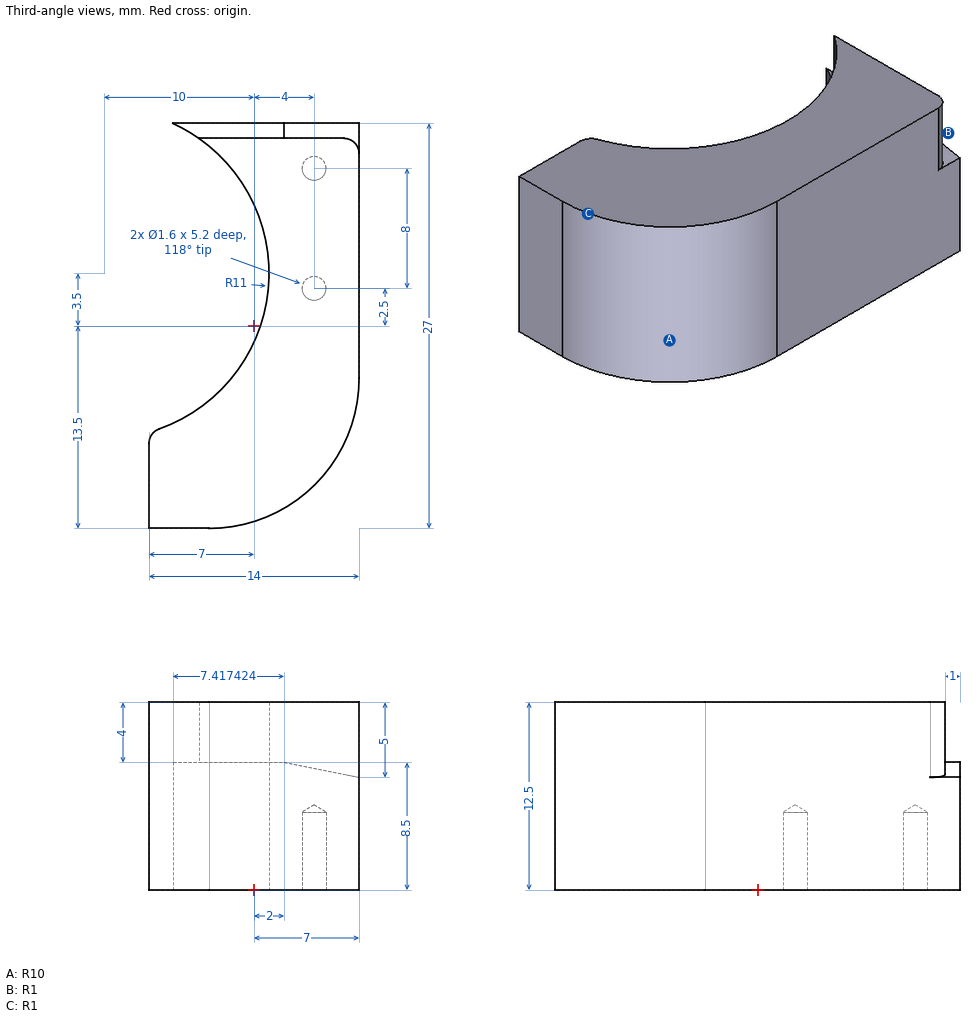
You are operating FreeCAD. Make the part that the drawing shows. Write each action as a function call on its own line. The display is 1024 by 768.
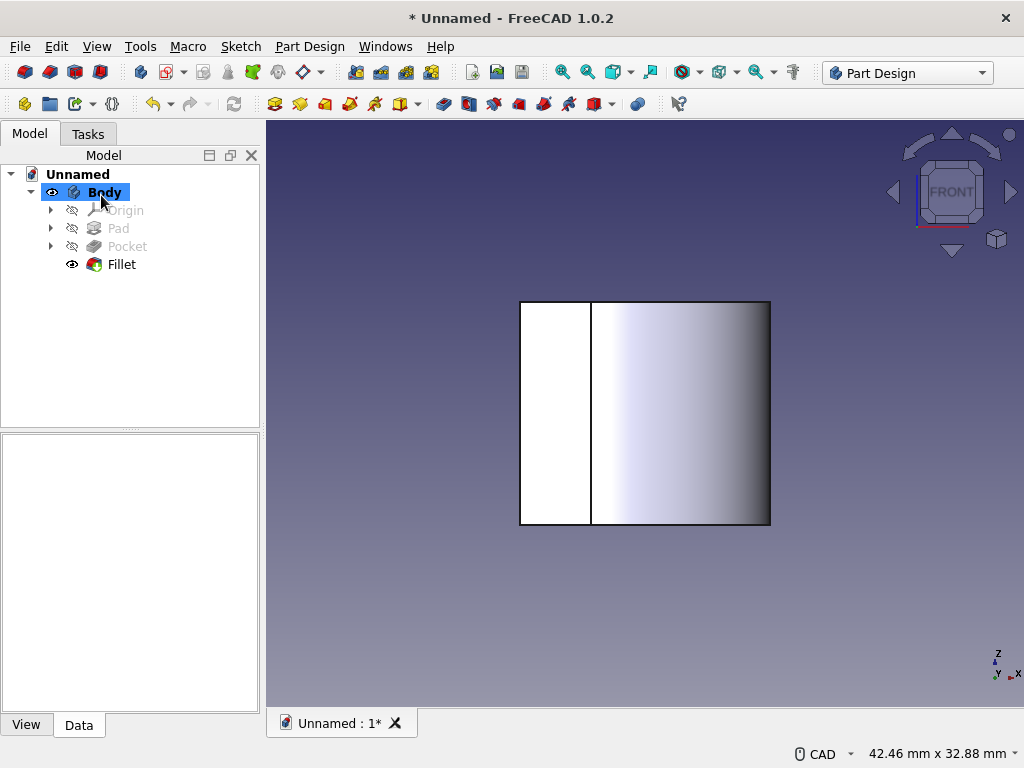
click(563, 72)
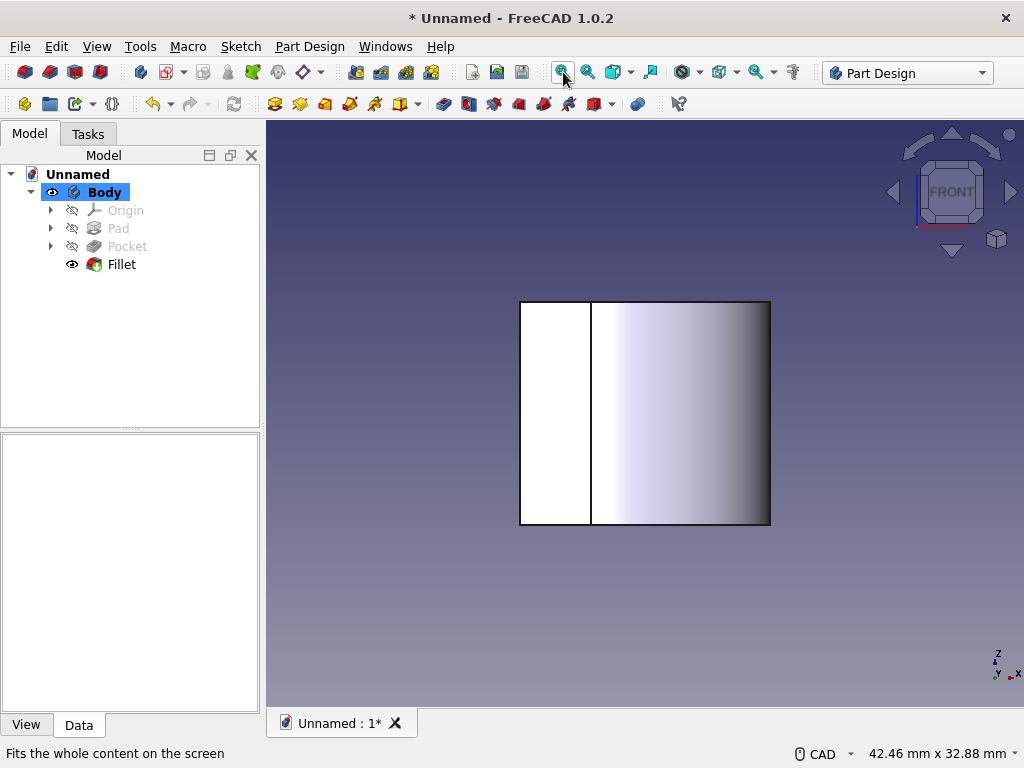
key(3)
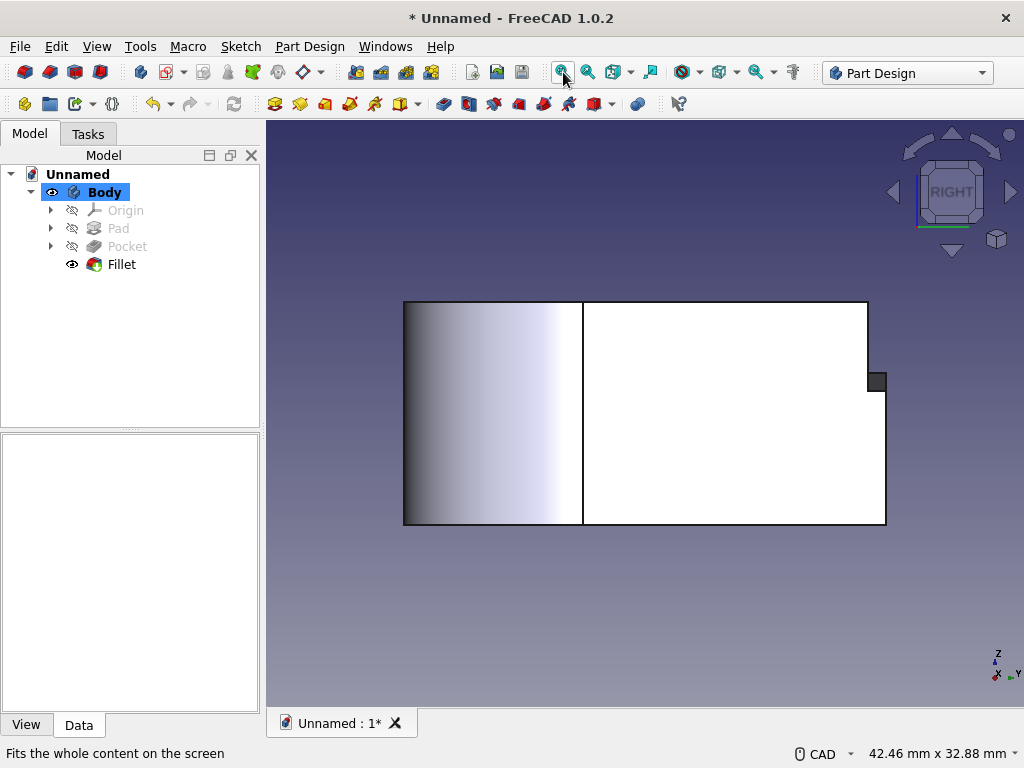
click(868, 346)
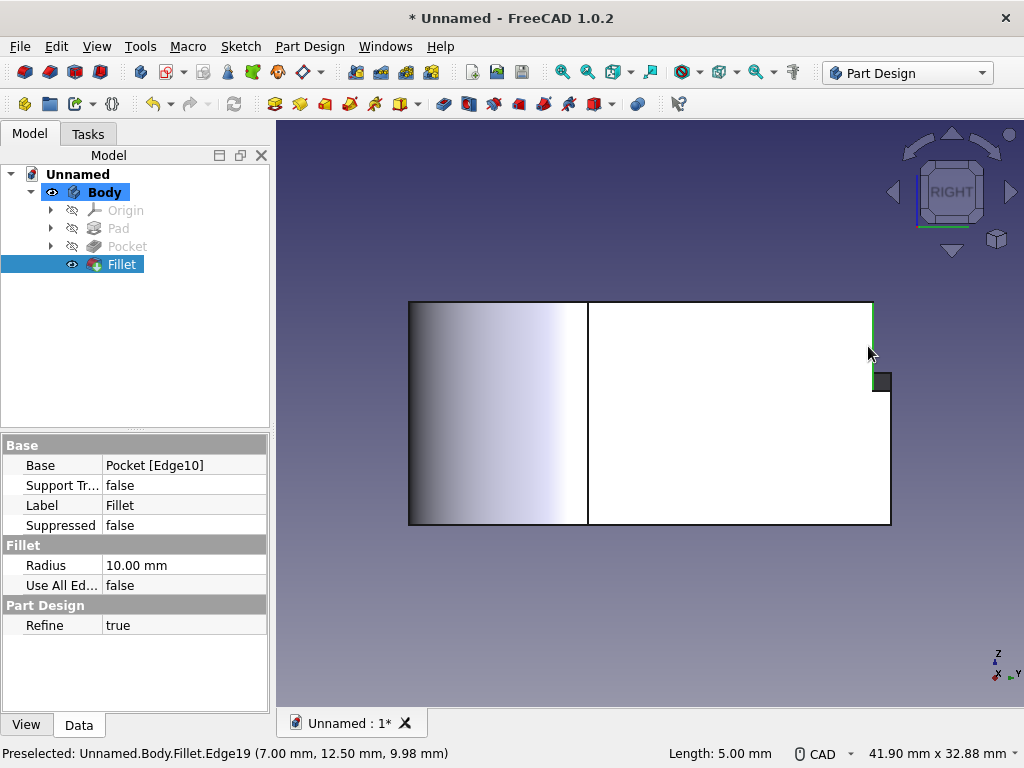
click(25, 72)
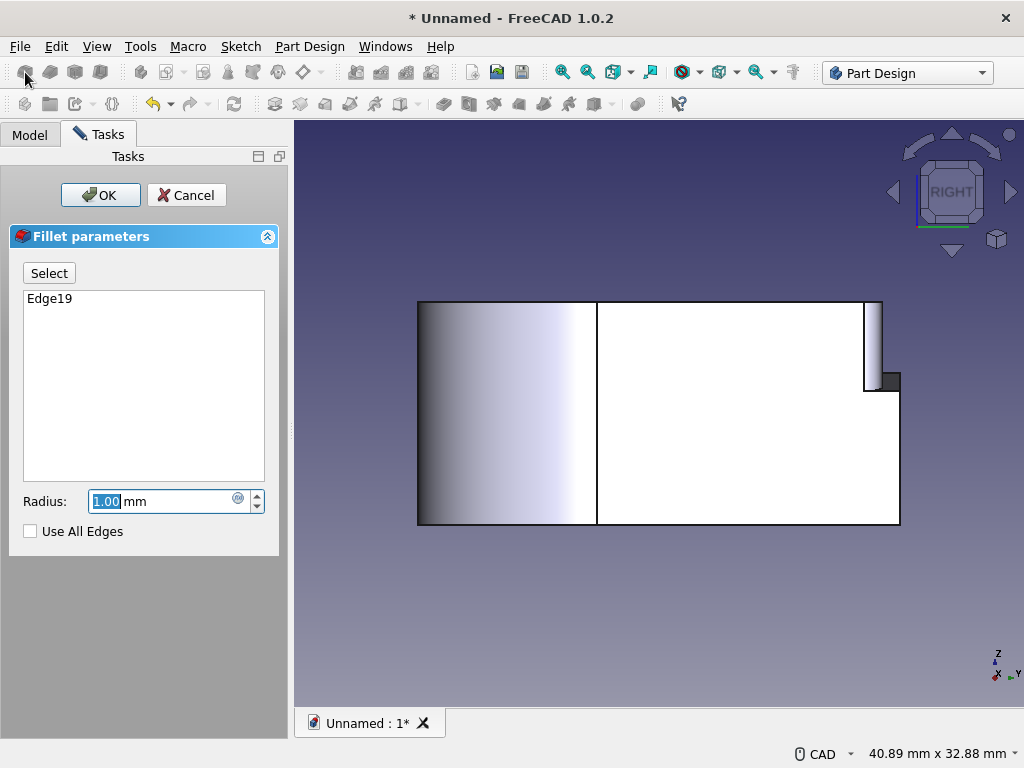
text(1)
key(Tab)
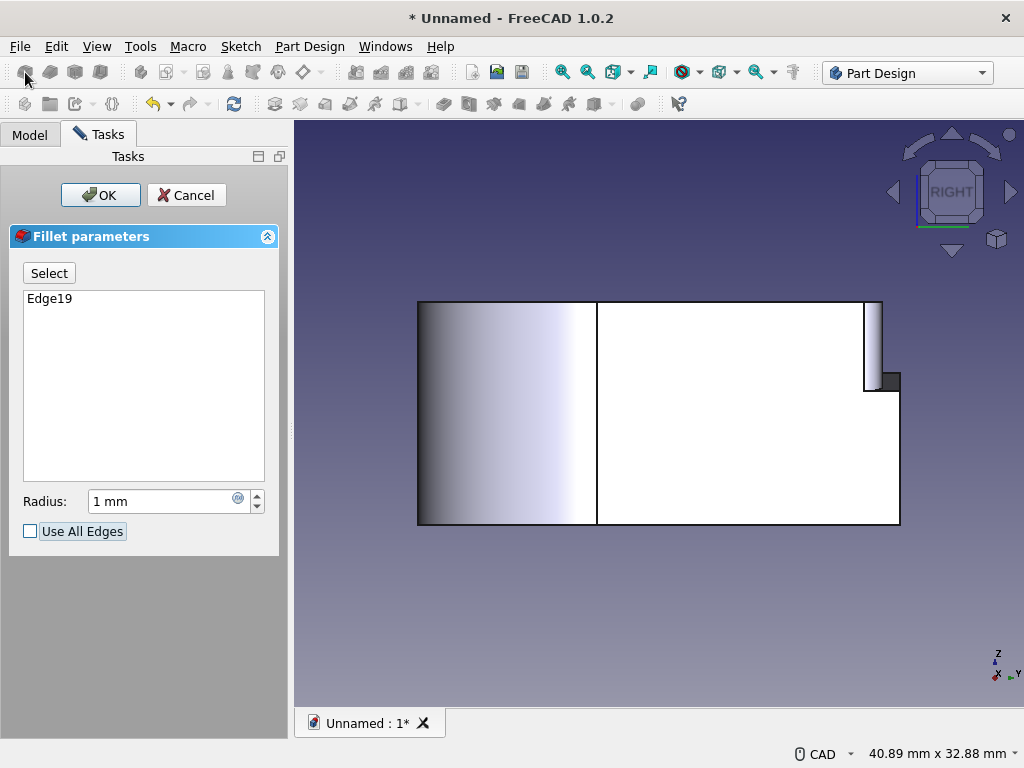
click(101, 195)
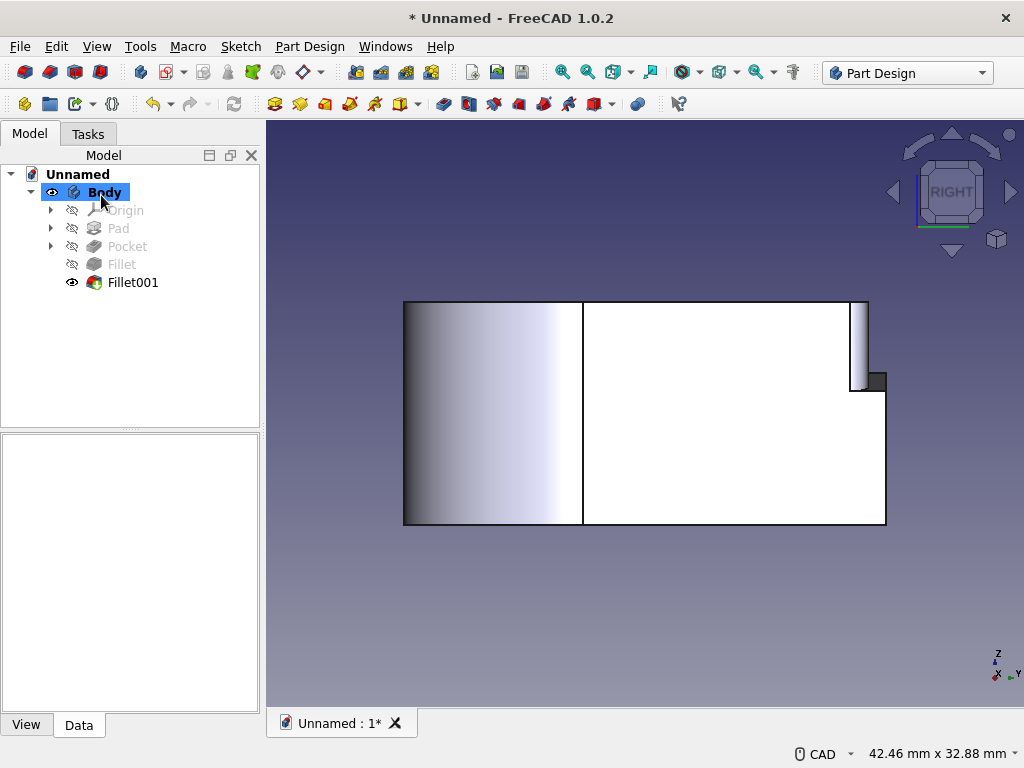
key(5)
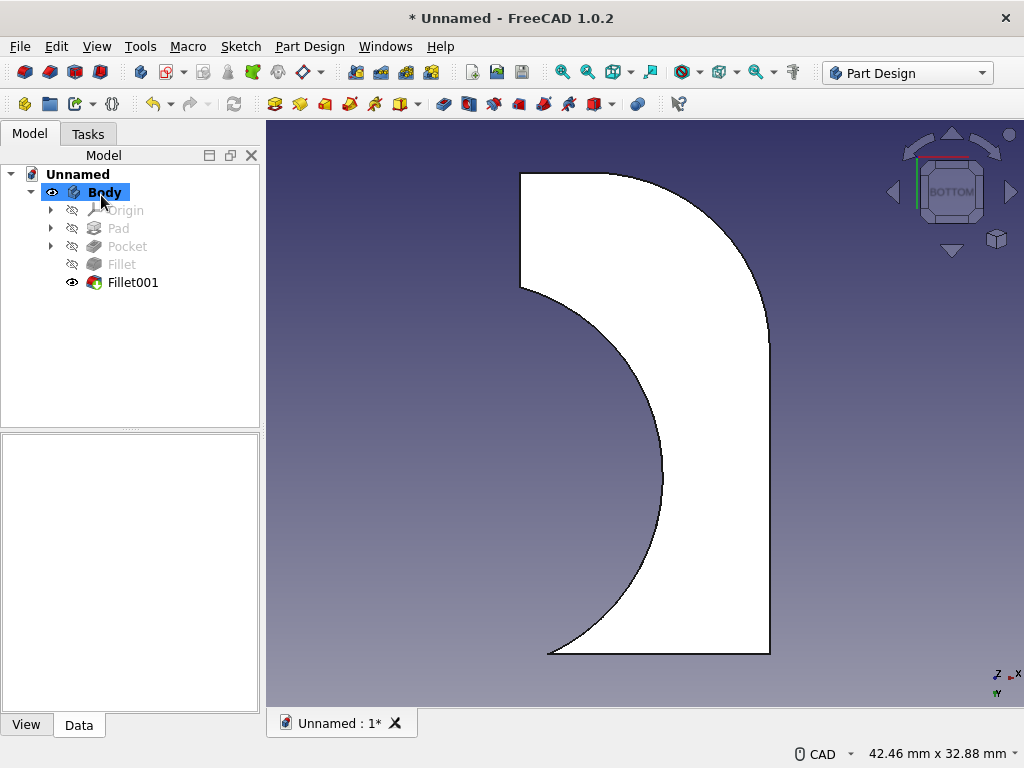
click(645, 275)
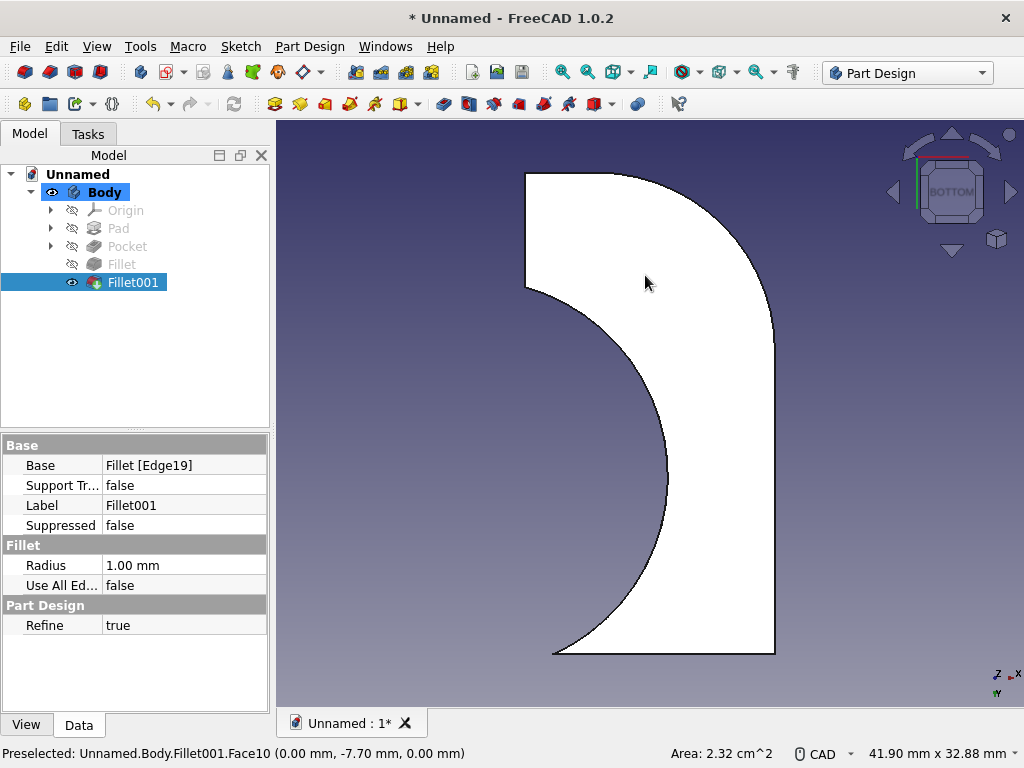
click(166, 72)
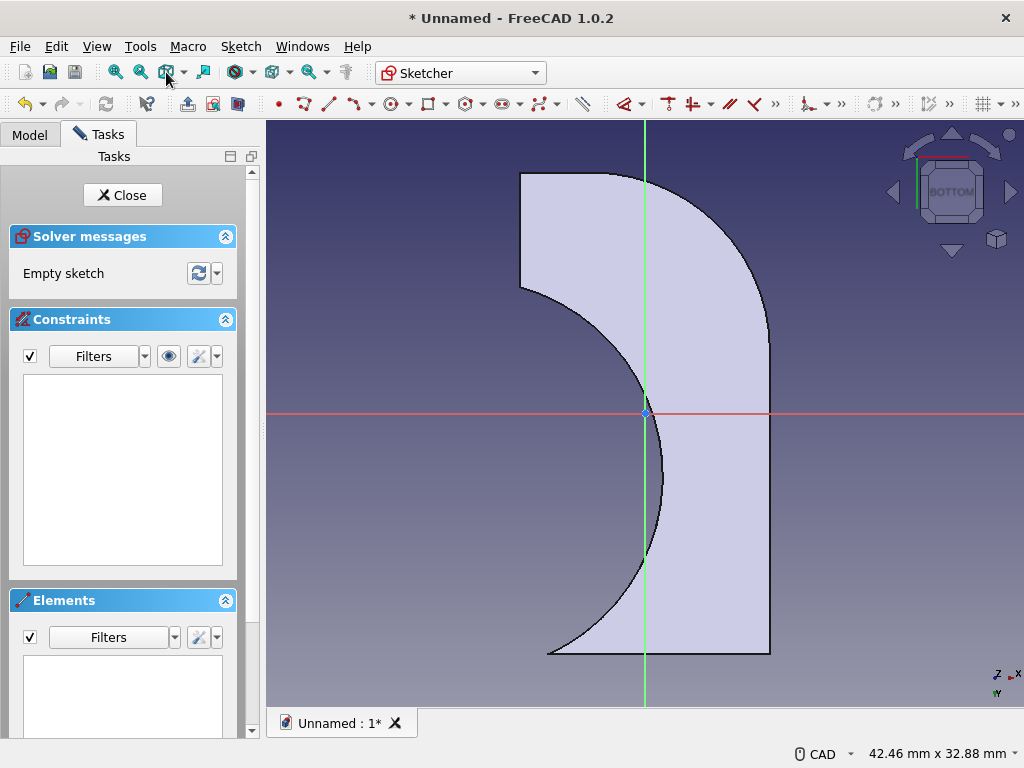
scroll(823, 637, up, 3)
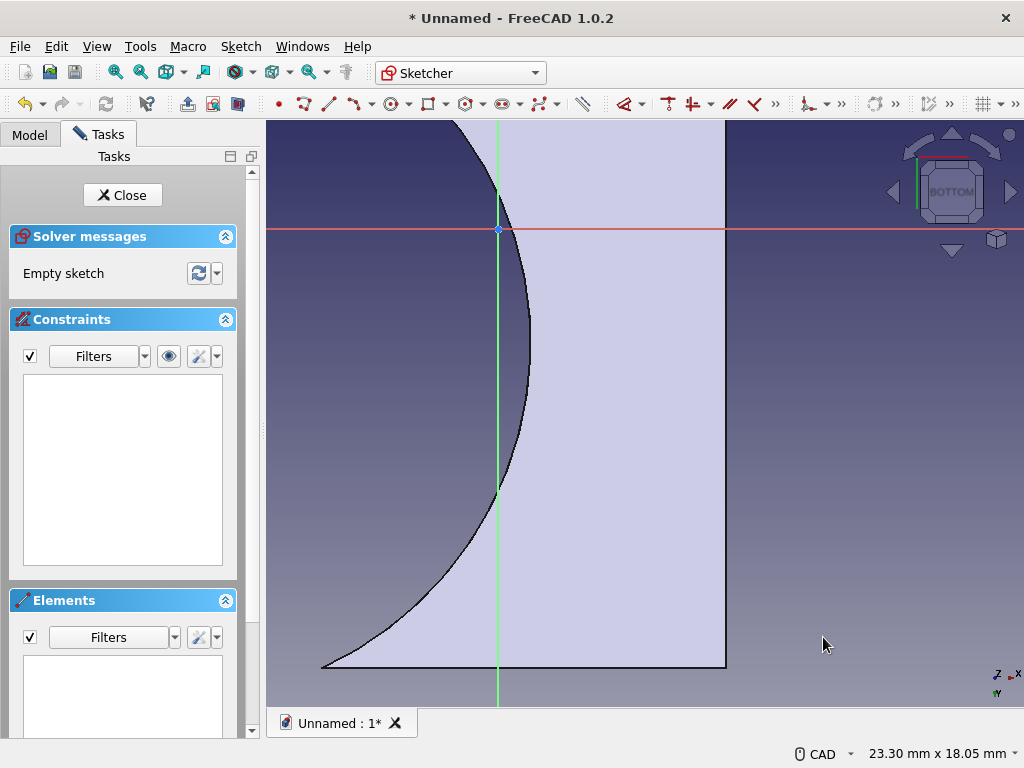
click(390, 104)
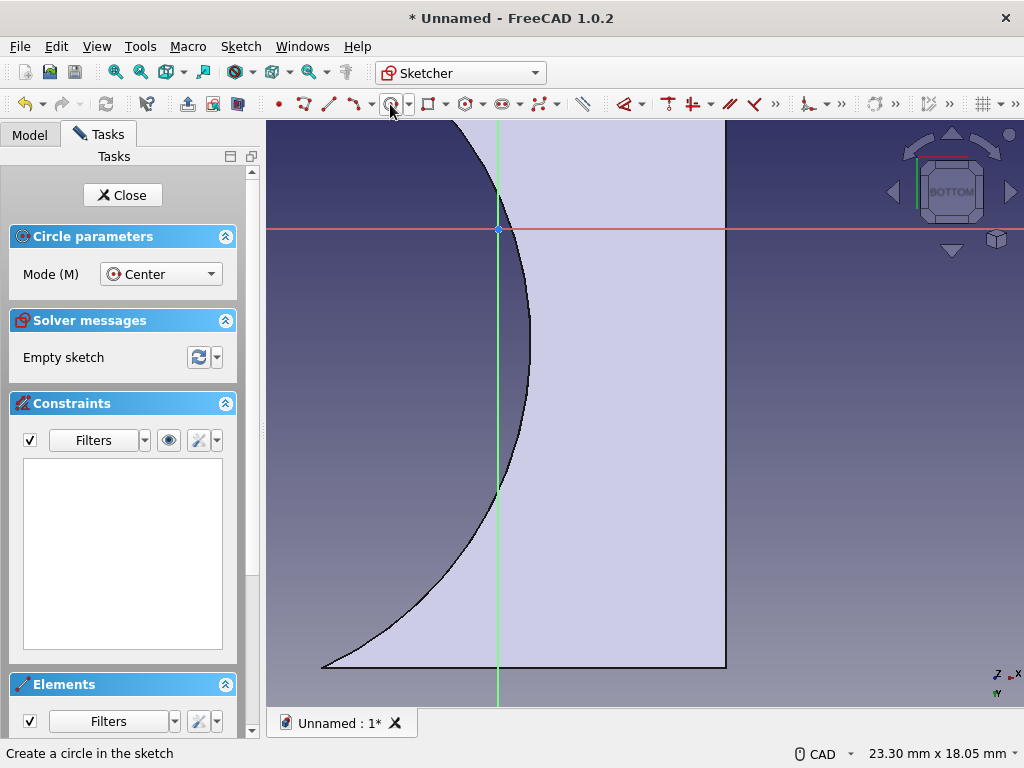
click(628, 310)
click(647, 292)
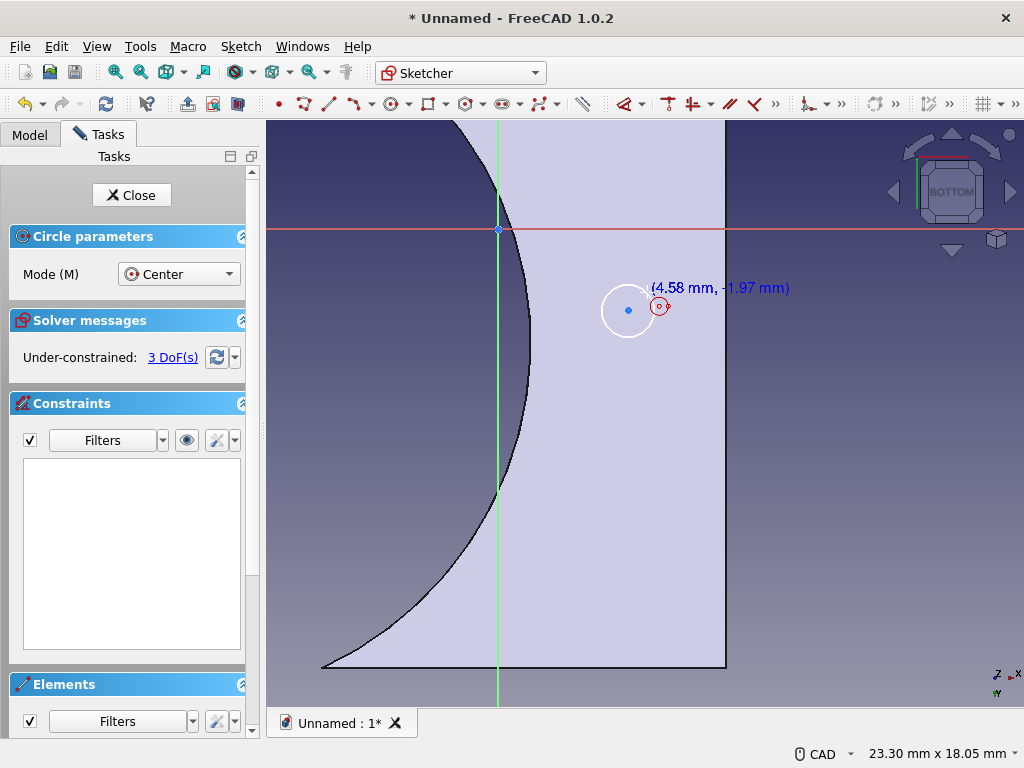
click(628, 571)
click(647, 552)
key(Escape)